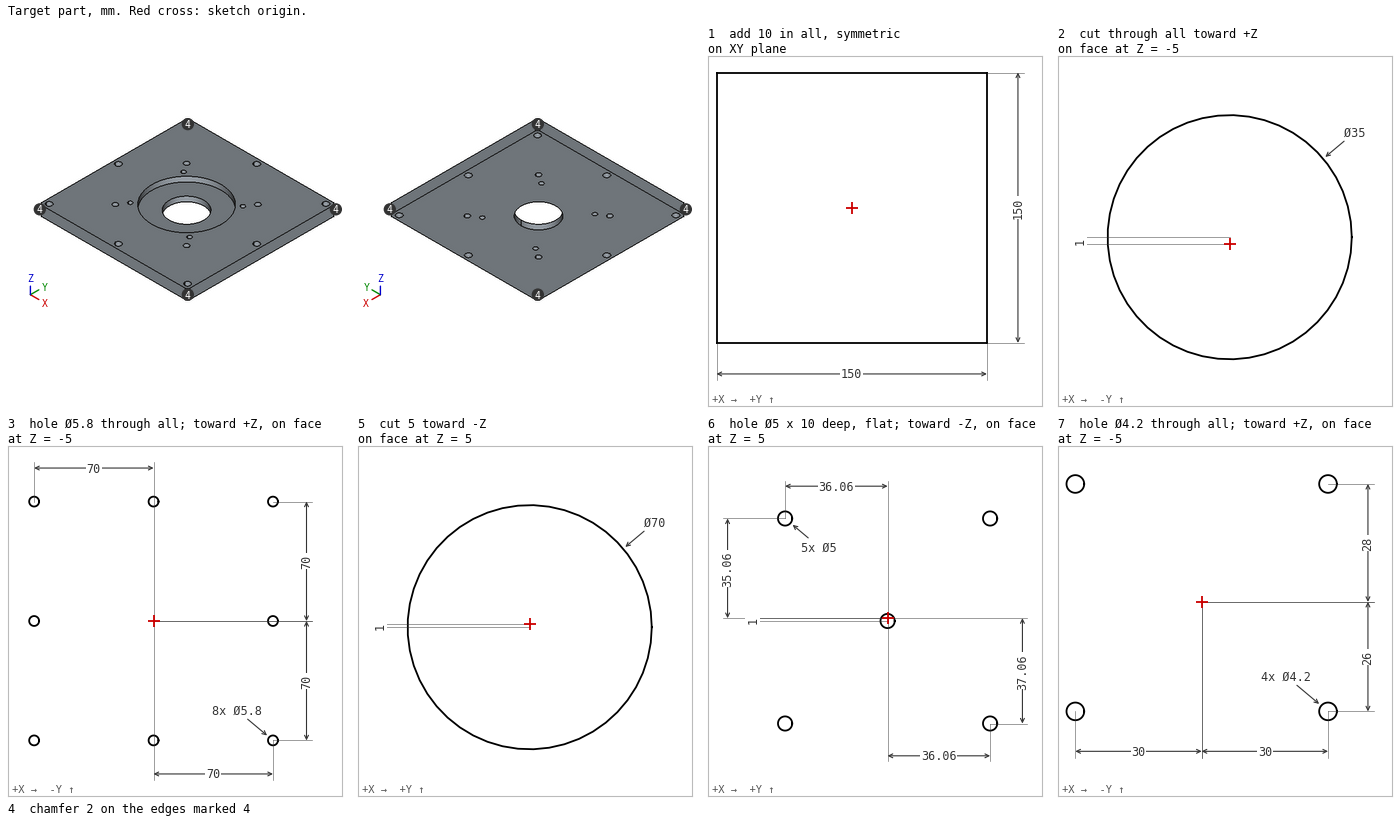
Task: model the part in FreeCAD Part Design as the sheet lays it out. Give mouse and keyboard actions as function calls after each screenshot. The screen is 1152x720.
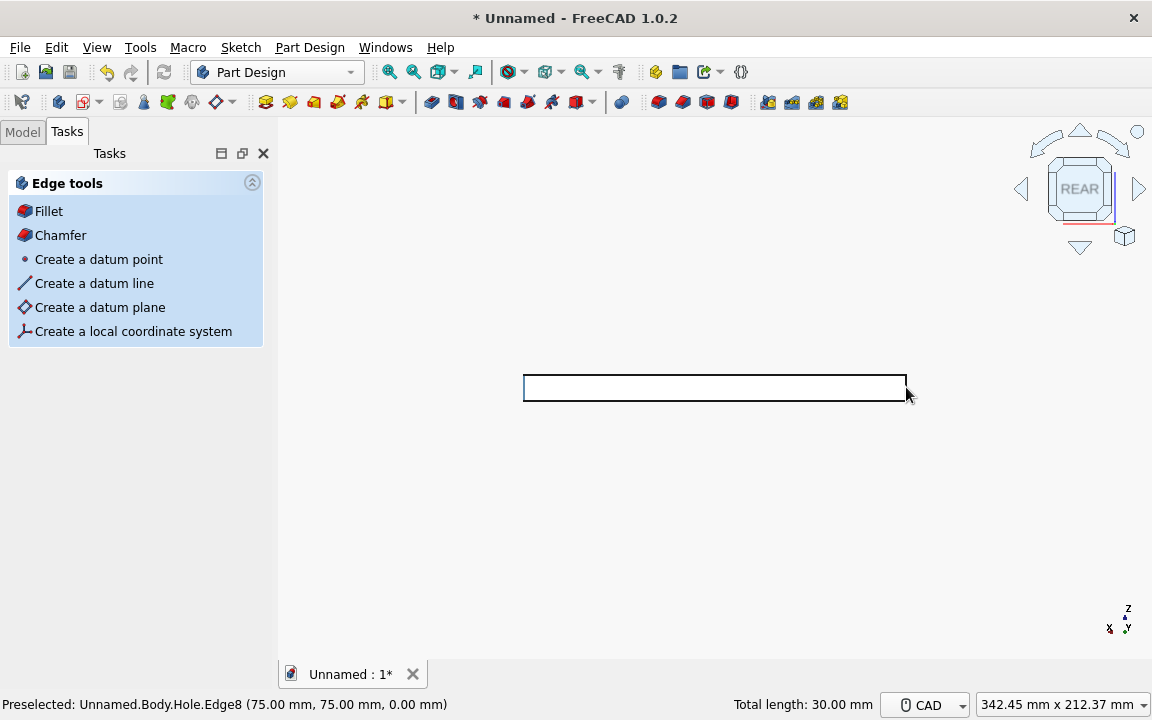
click(906, 387, ctrl)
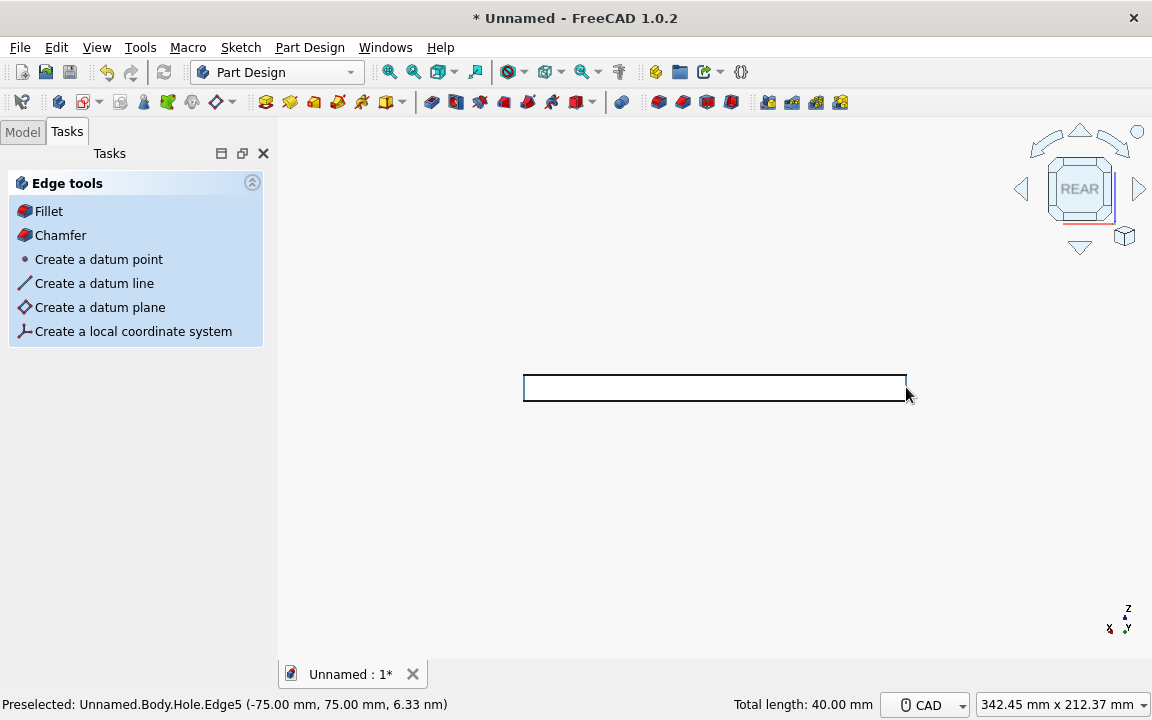
click(684, 102)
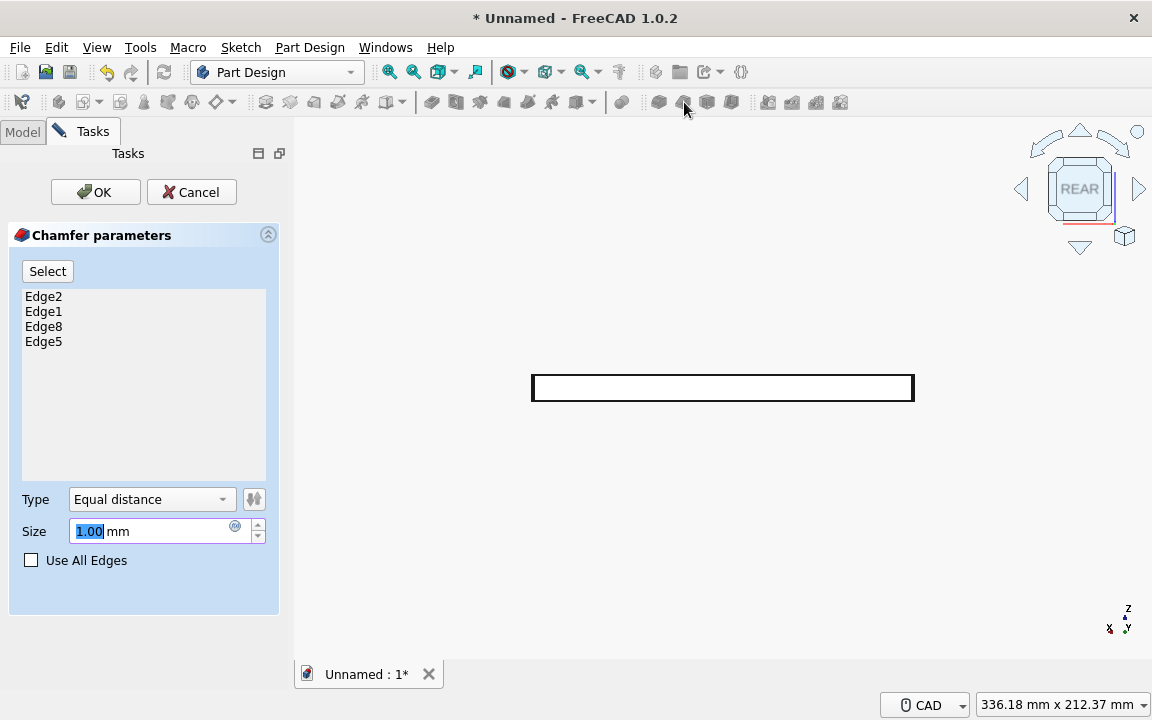
text(2)
key(Tab)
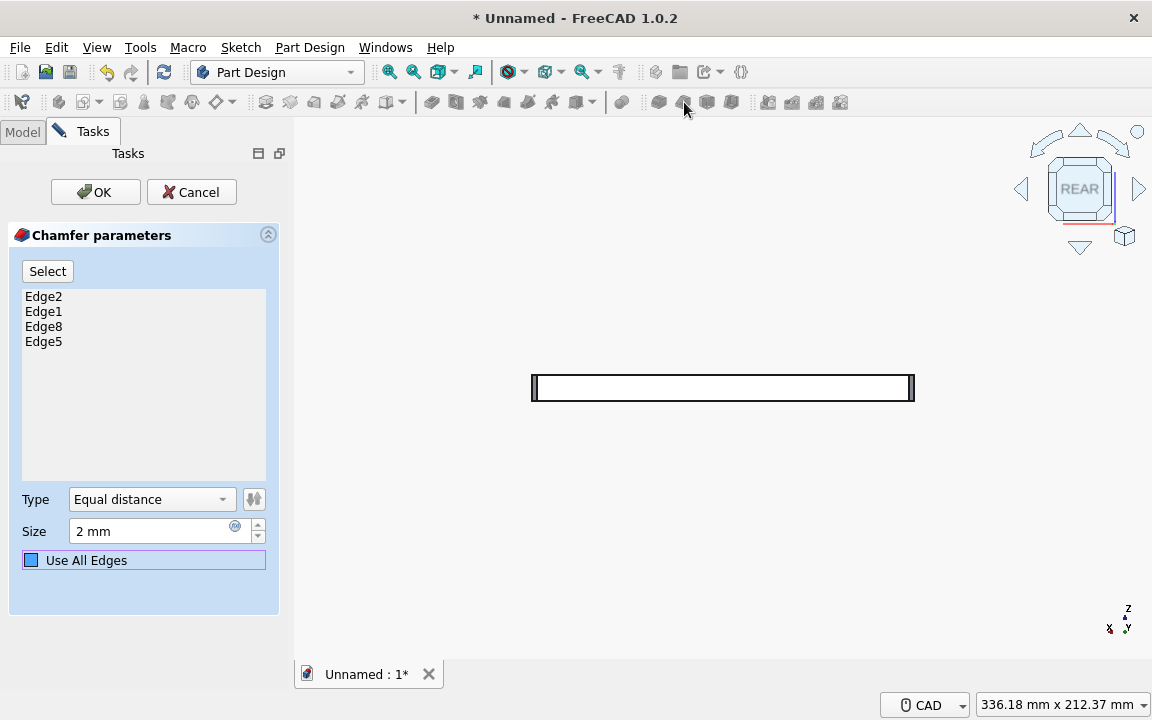
click(96, 192)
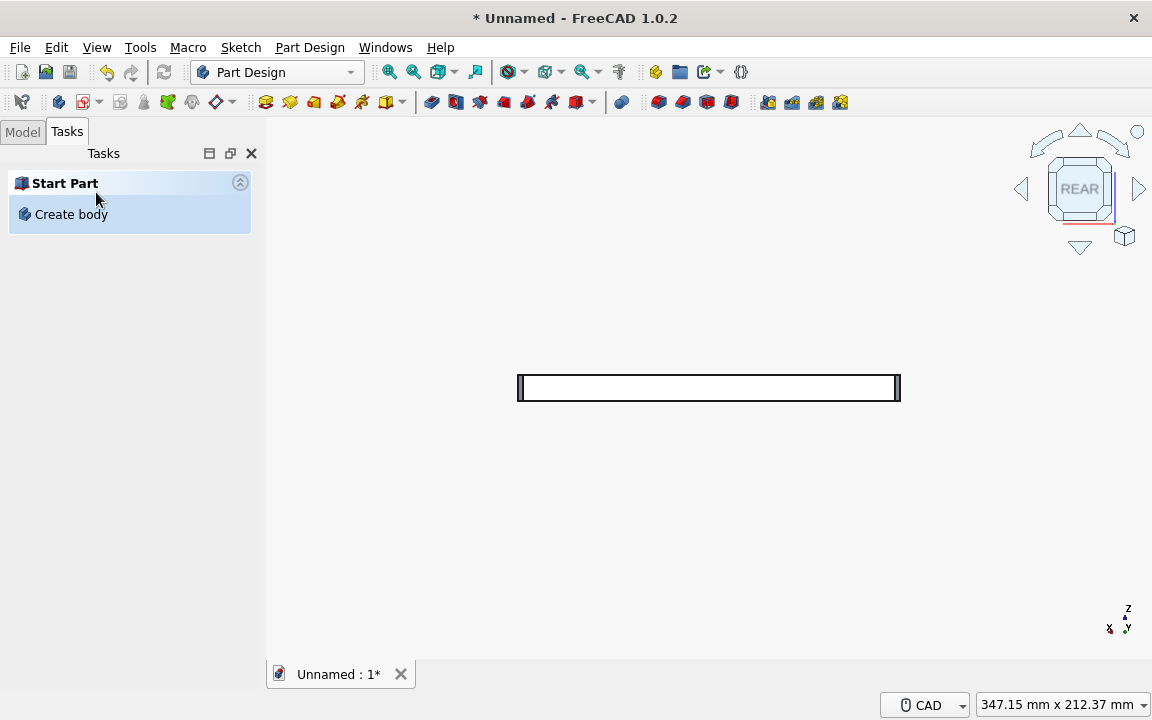
key(v)
key(f)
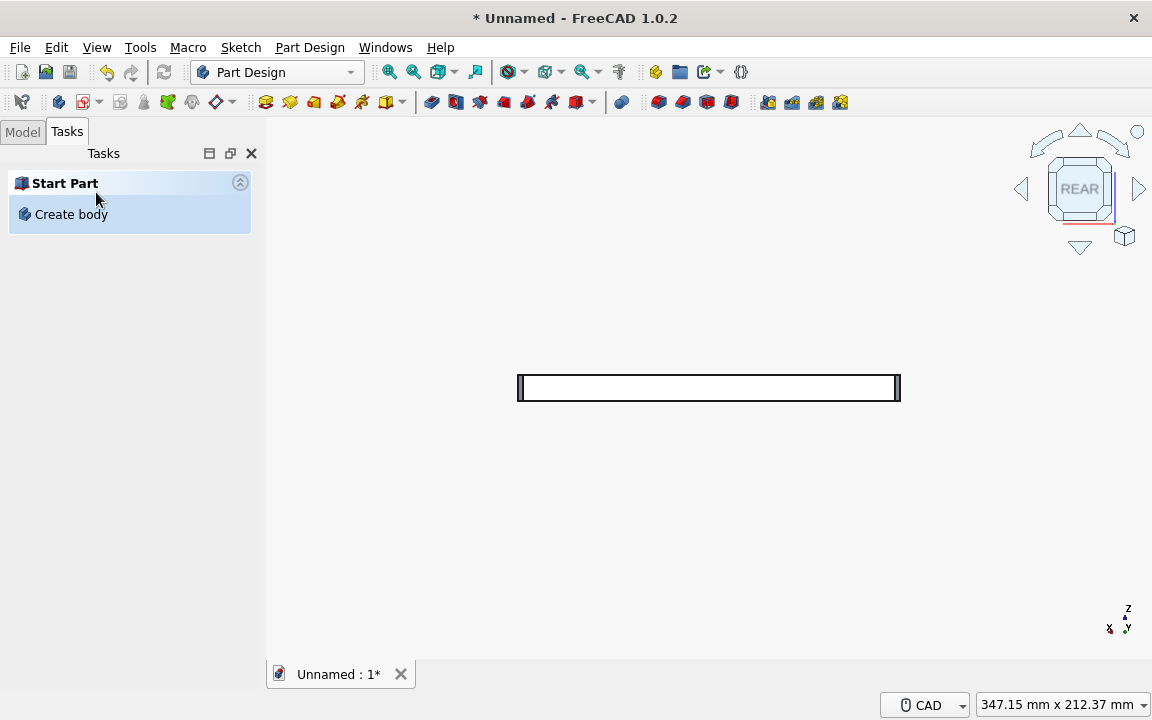
key(0)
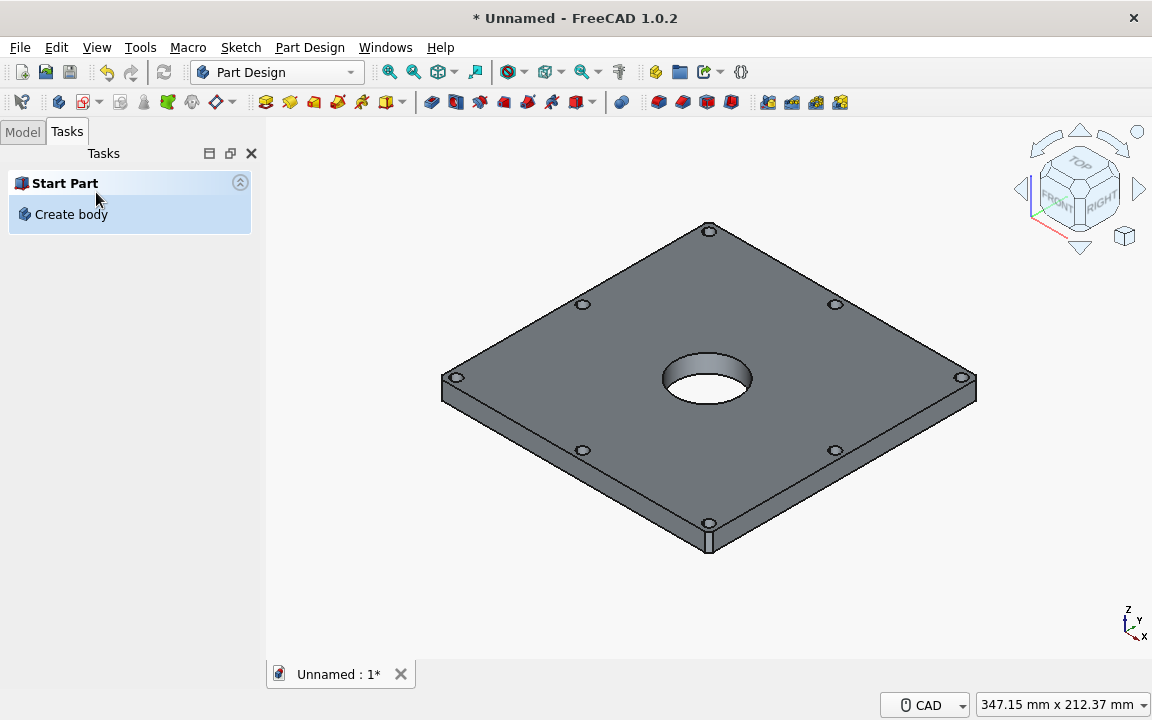
click(554, 377)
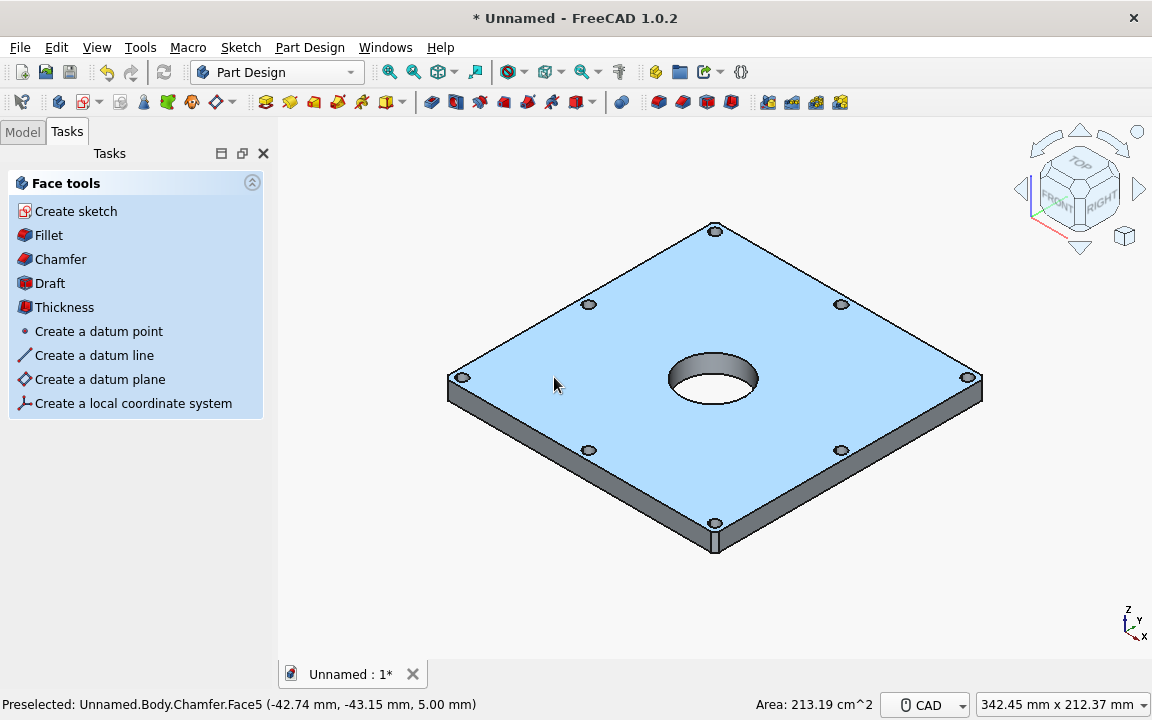
click(84, 102)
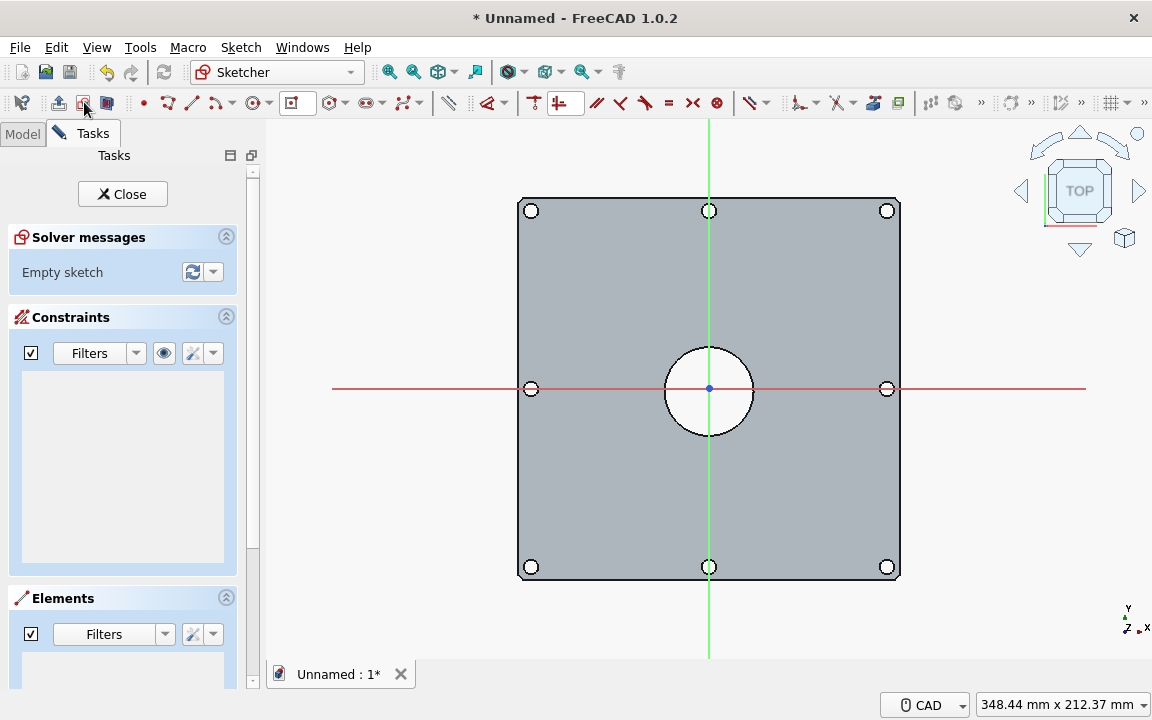
scroll(792, 395, up, 3)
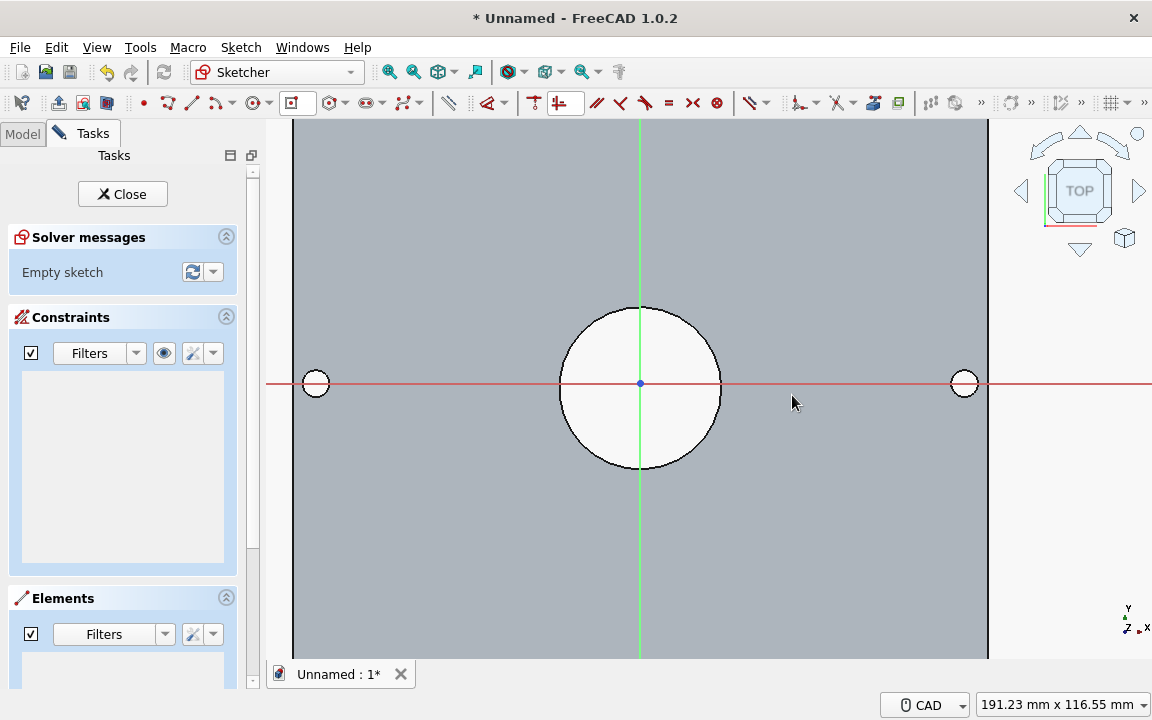
key(g)
key(c)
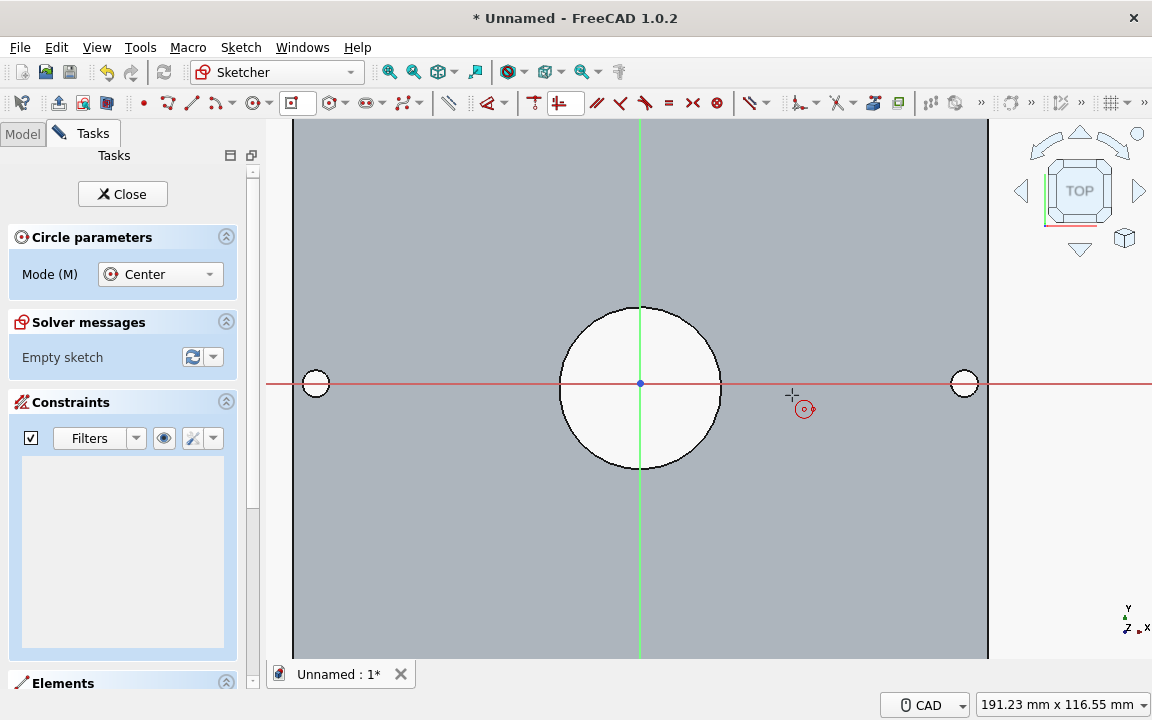
scroll(640, 388, up, 7)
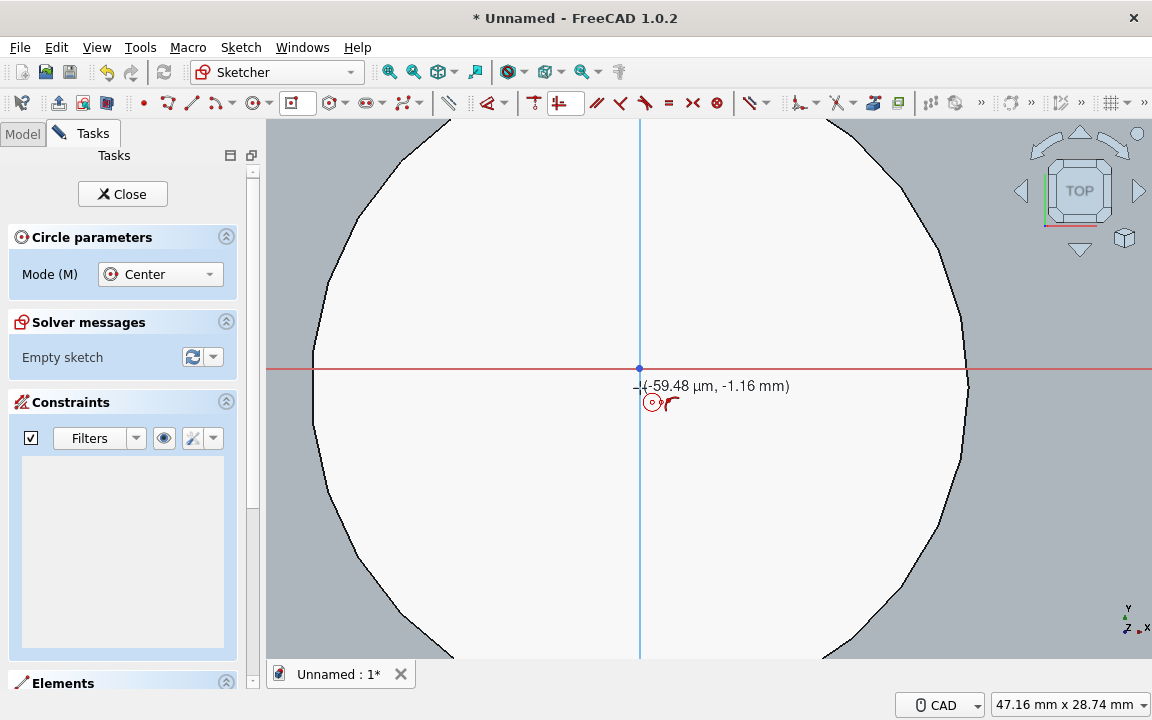
click(640, 388)